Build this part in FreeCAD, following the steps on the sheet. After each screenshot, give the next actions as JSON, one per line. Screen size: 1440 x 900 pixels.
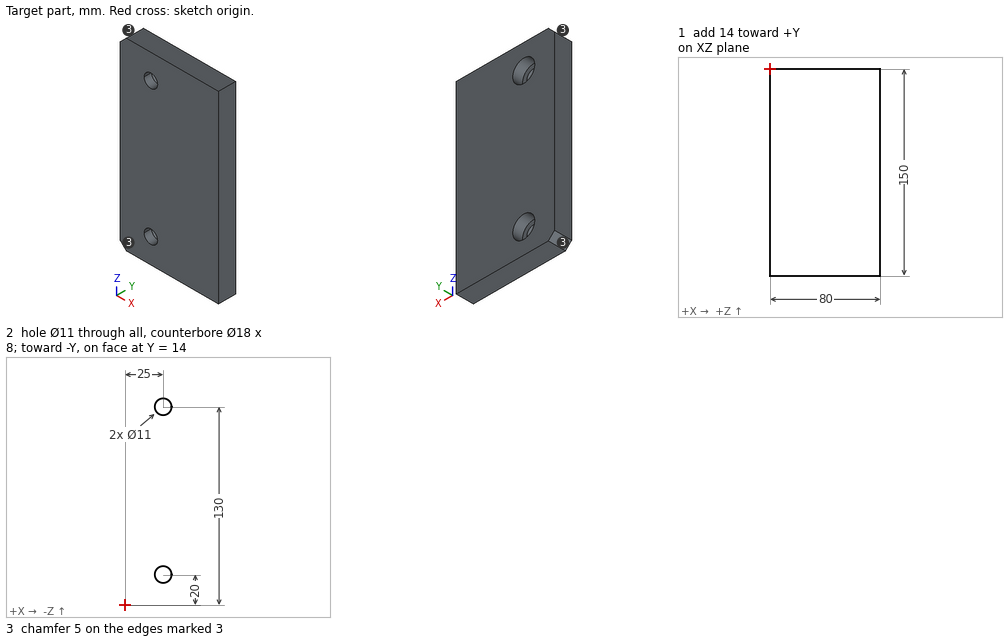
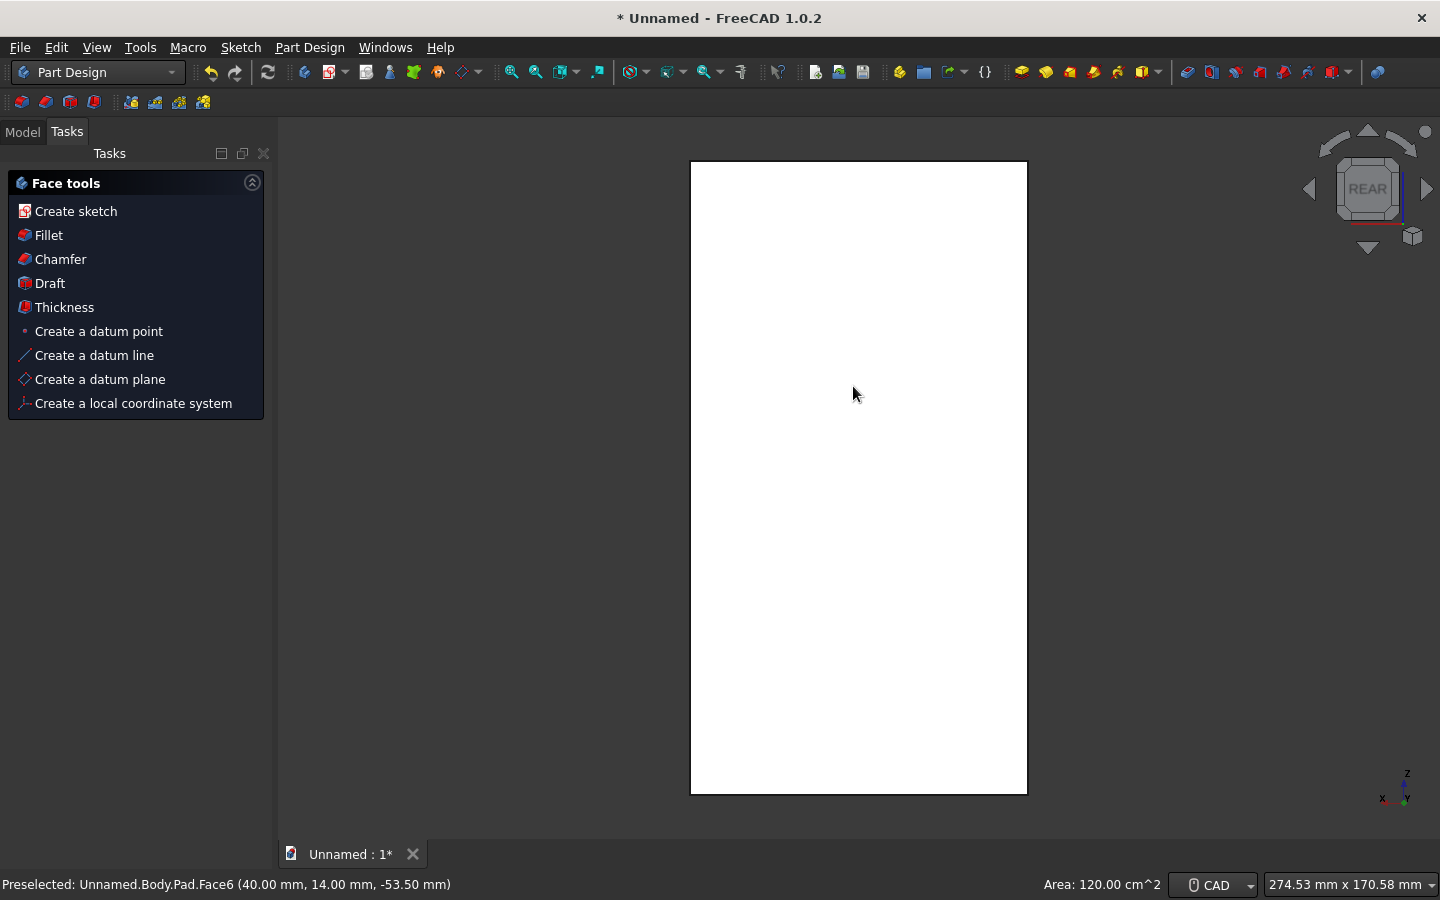
{"action": "left_click", "coordinate": [330, 72]}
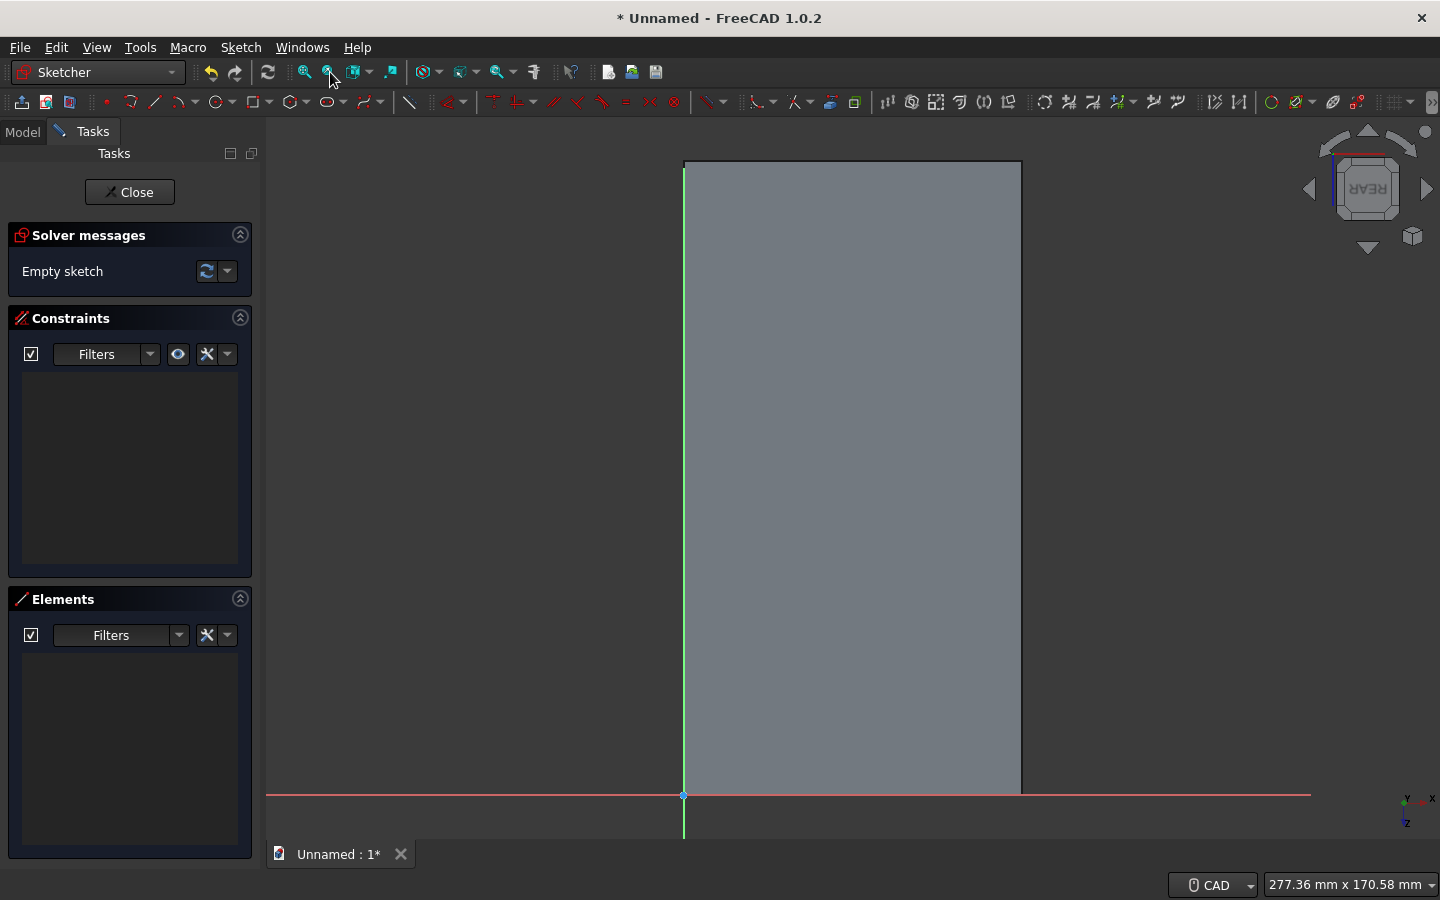
{"action": "scroll", "coordinate": [948, 339], "scroll_direction": "down", "scroll_amount": 1}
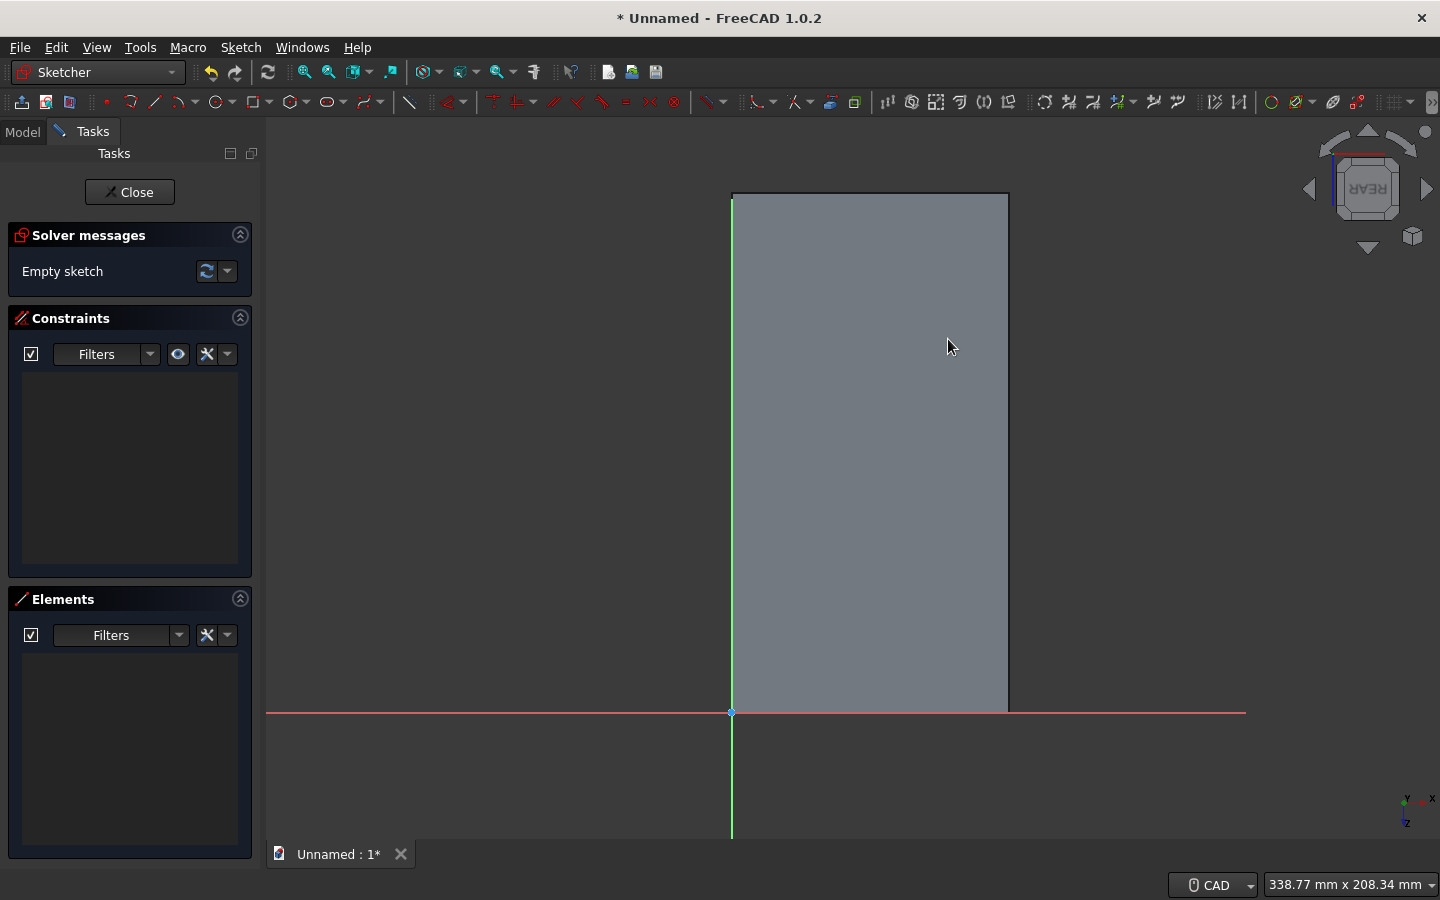
{"action": "left_click", "coordinate": [216, 102]}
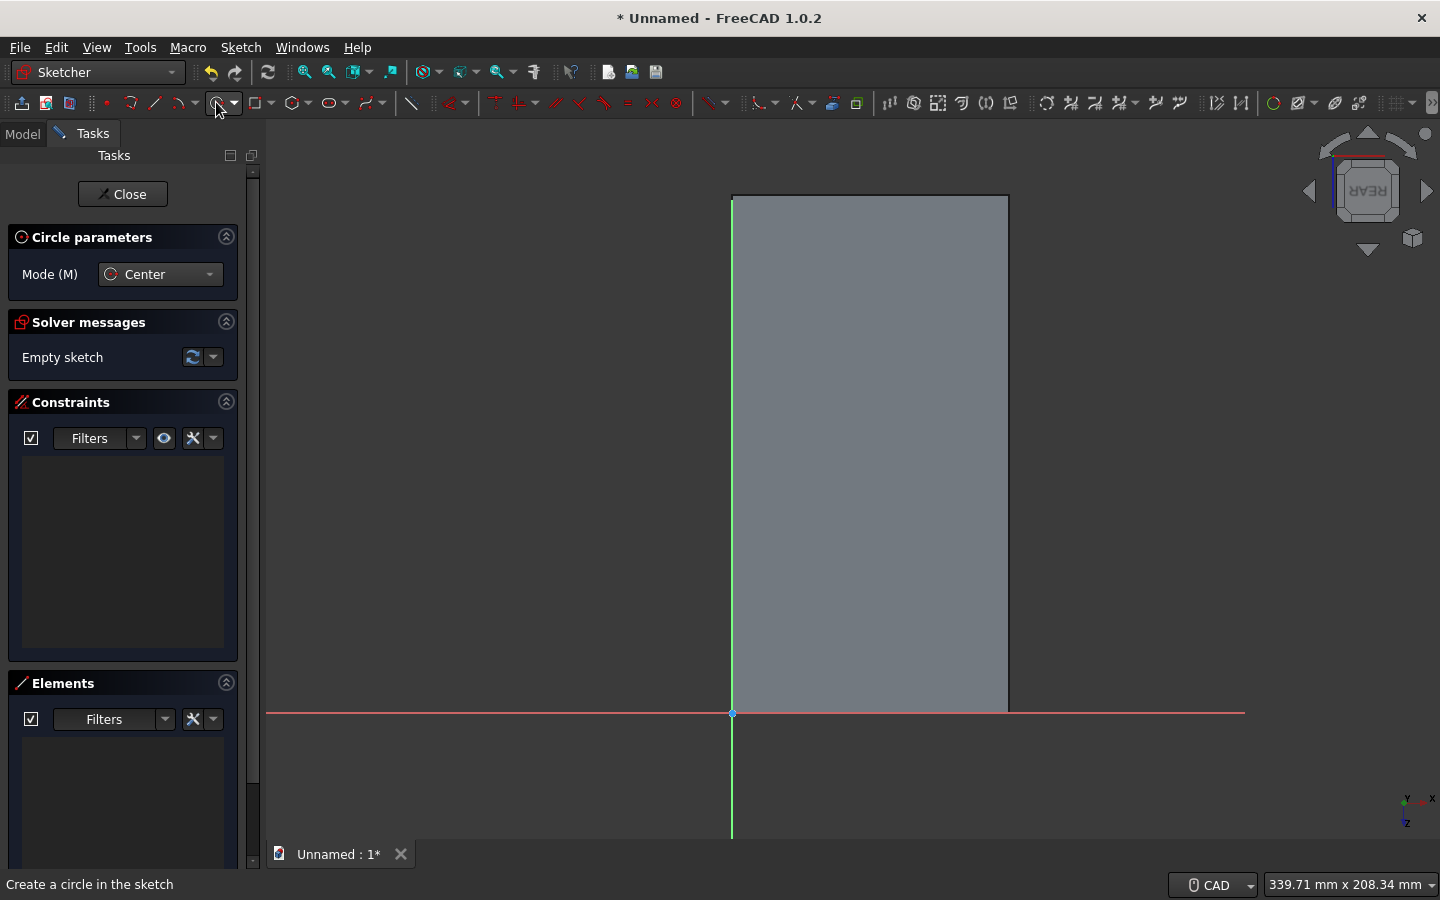
{"action": "left_click", "coordinate": [818, 264]}
{"action": "mouse_move", "coordinate": [832, 250]}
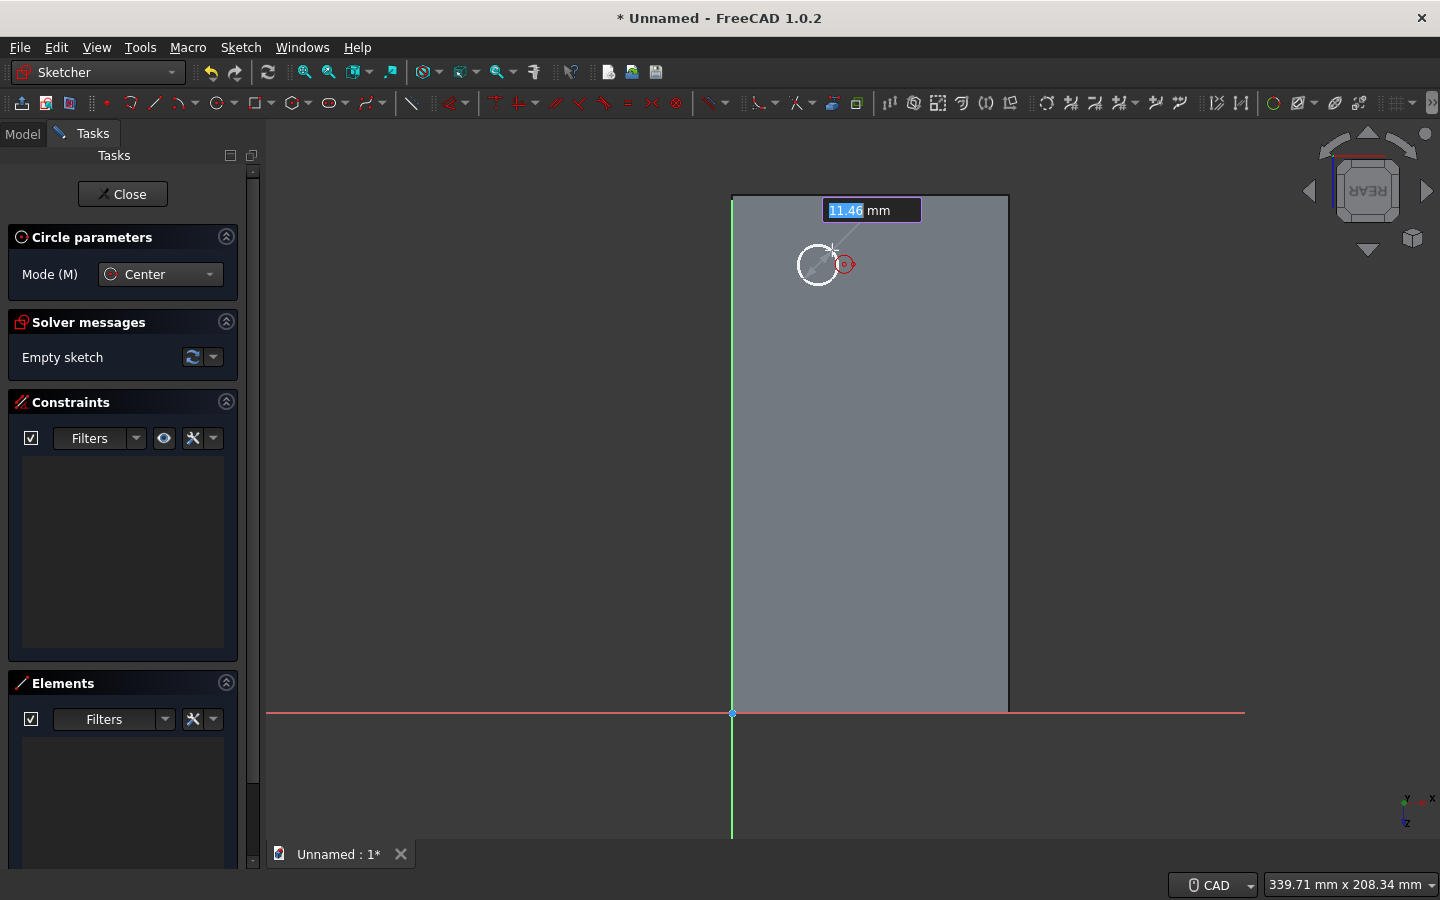
{"action": "type", "text": "11"}
{"action": "key", "text": "Return"}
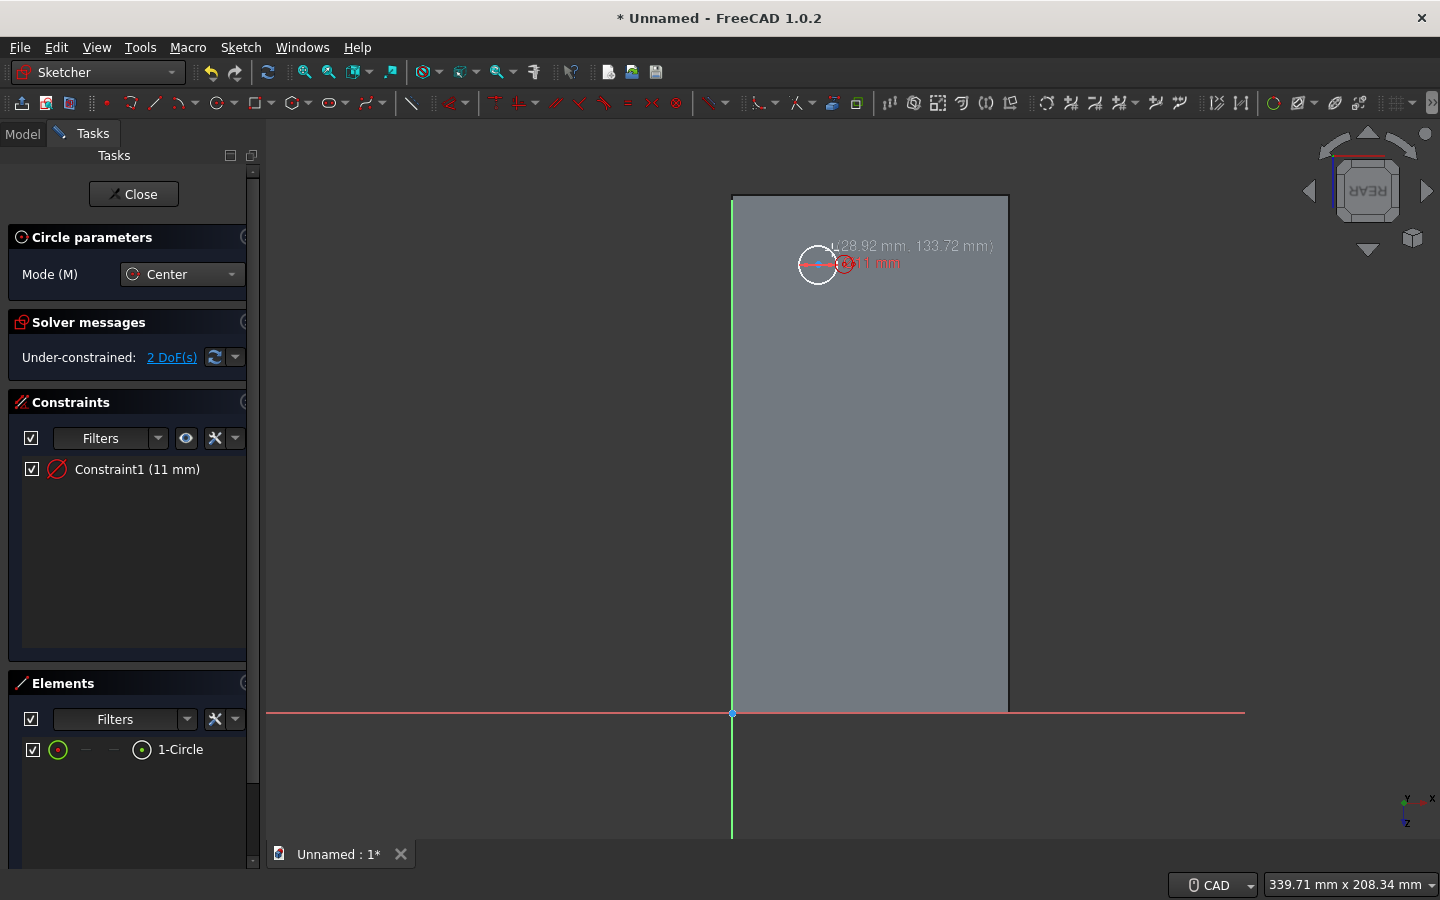
{"action": "left_click", "coordinate": [818, 644]}
{"action": "mouse_move", "coordinate": [832, 631]}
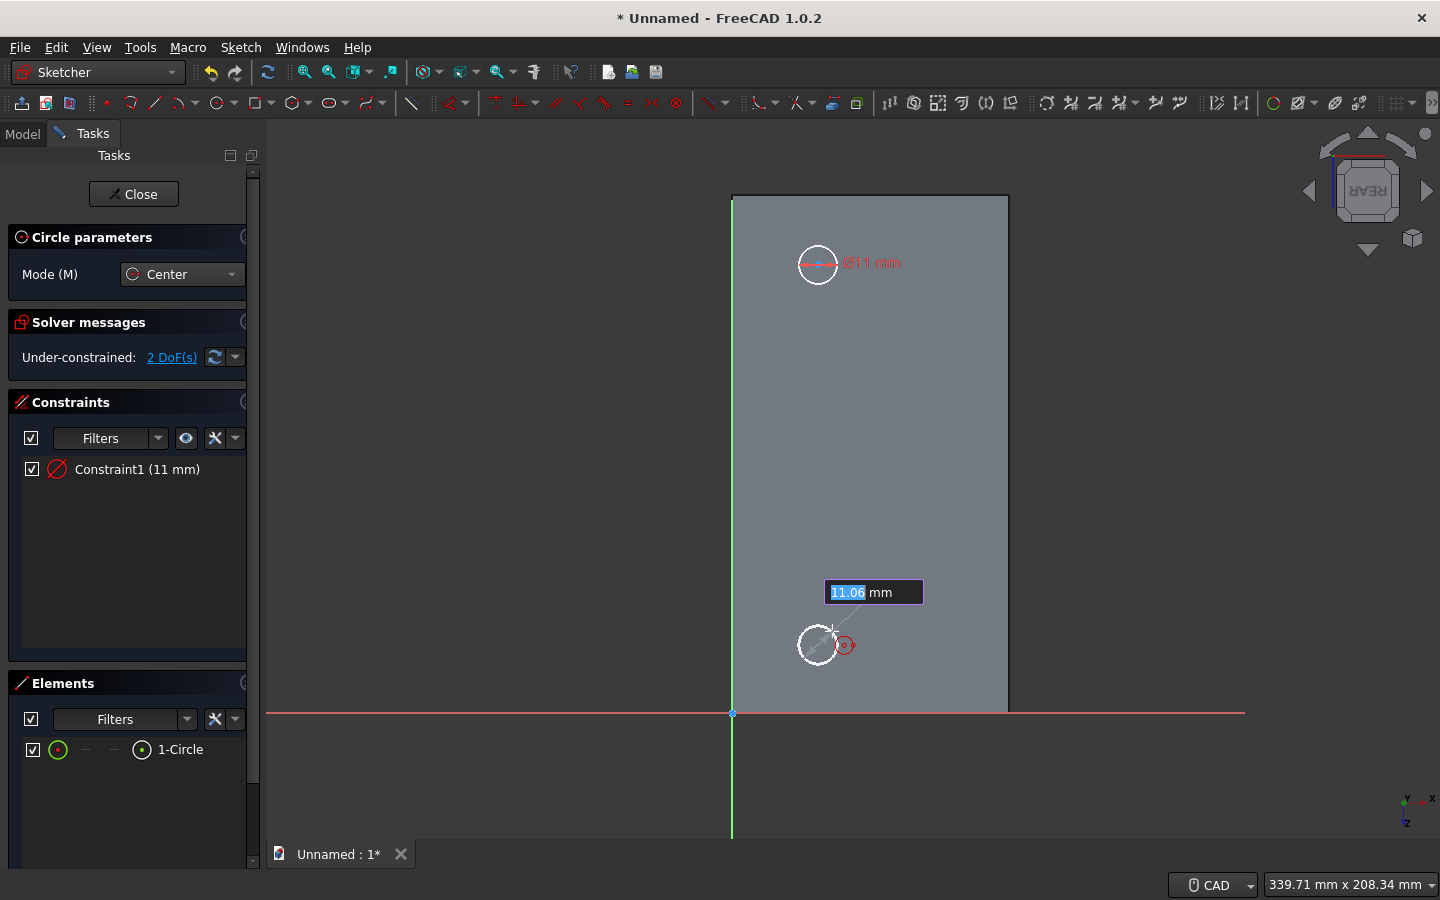
{"action": "type", "text": "11"}
{"action": "key", "text": "Return"}
{"action": "key", "text": "Escape"}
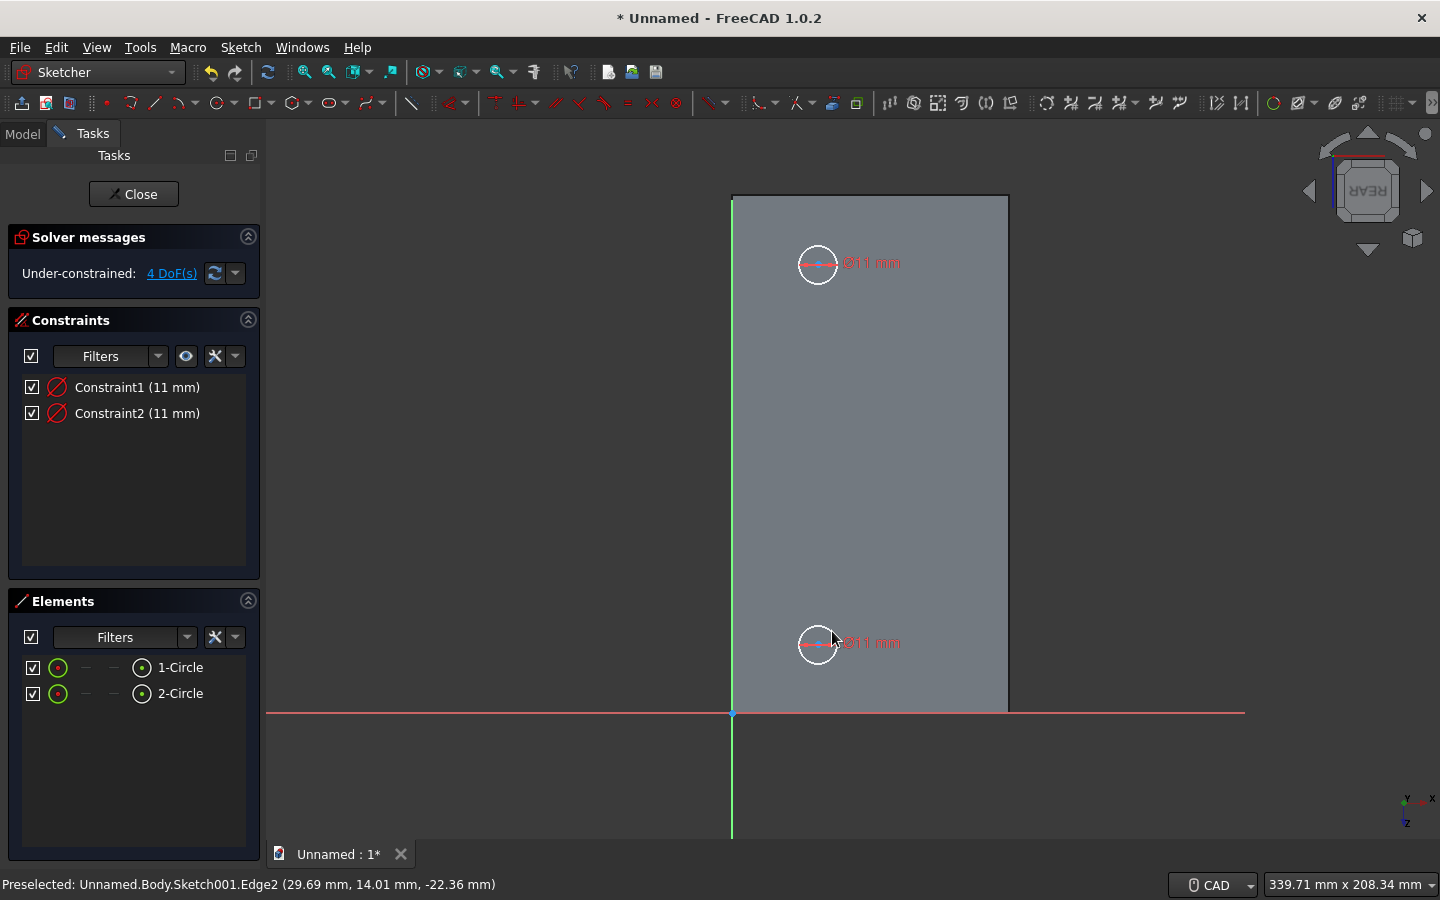
{"action": "left_click", "coordinate": [818, 265]}